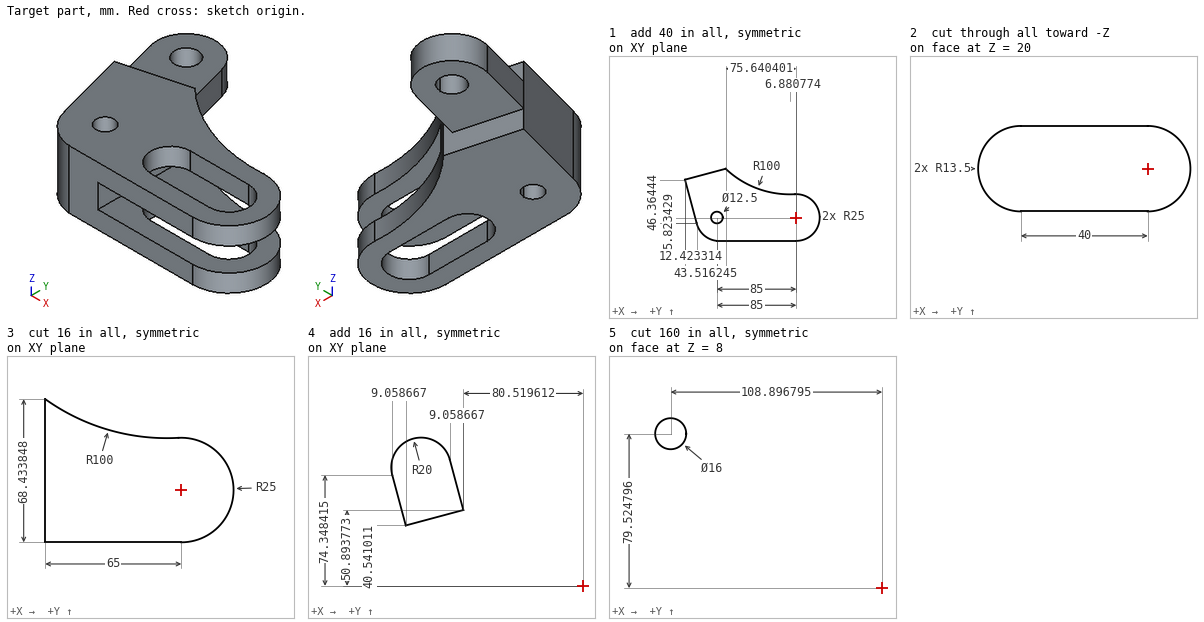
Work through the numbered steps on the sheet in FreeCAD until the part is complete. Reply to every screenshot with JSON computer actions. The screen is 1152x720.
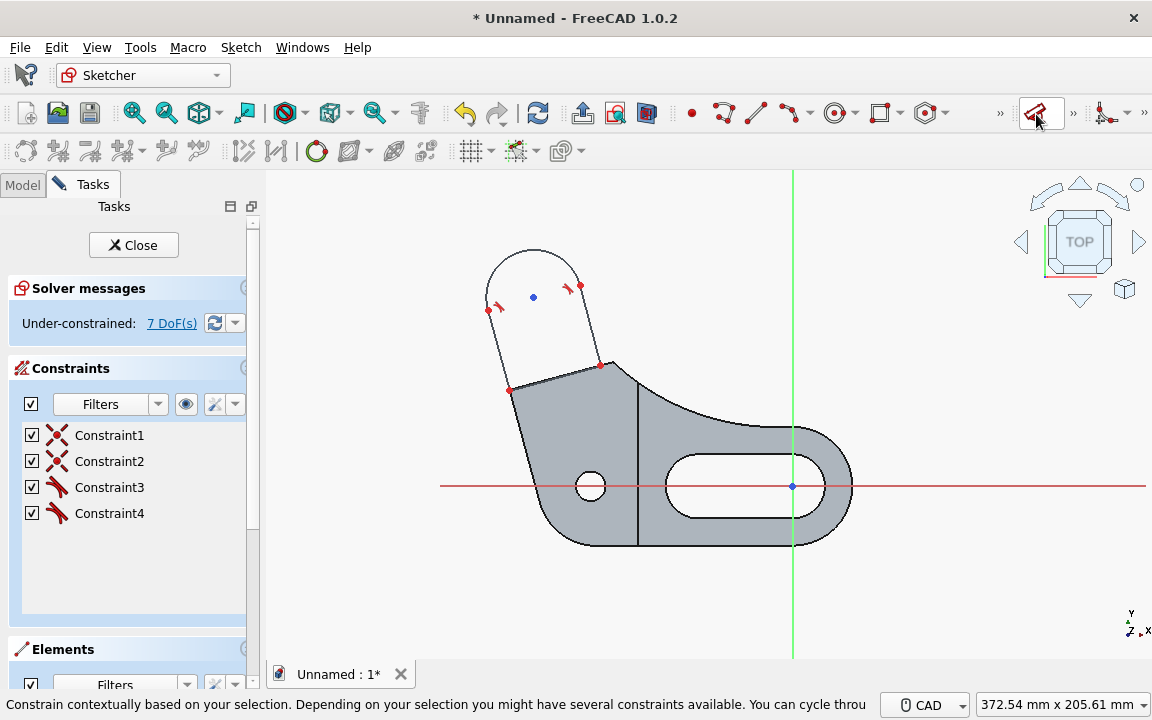
{"action": "left_click", "coordinate": [551, 253]}
{"action": "left_click", "coordinate": [562, 223]}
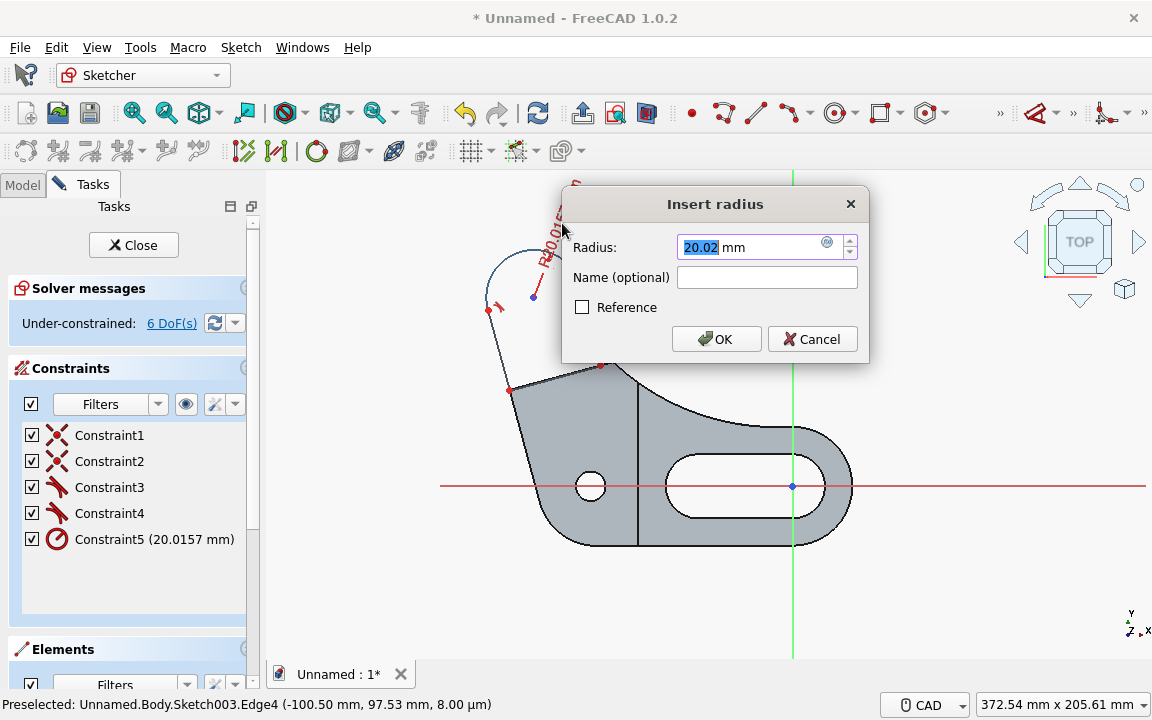
{"action": "type", "text": "20"}
{"action": "key", "text": "Return"}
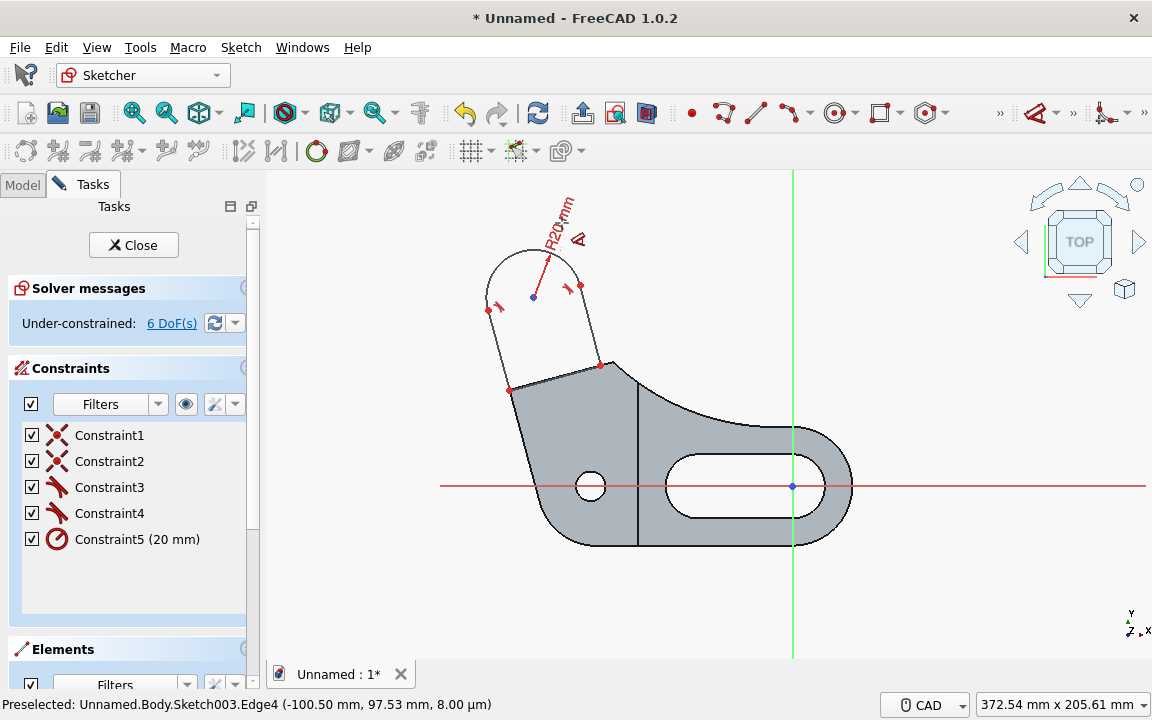
{"action": "scroll", "coordinate": [495, 334], "scroll_direction": "up", "scroll_amount": 4}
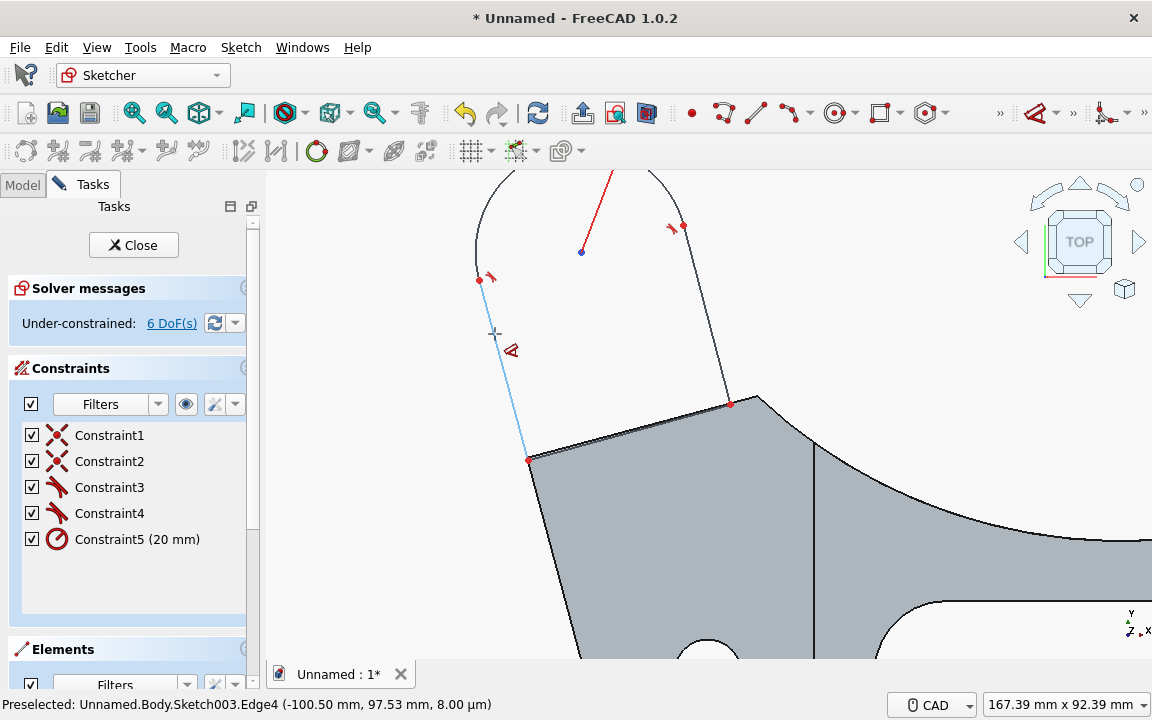
{"action": "left_click", "coordinate": [494, 334]}
{"action": "left_click", "coordinate": [504, 246]}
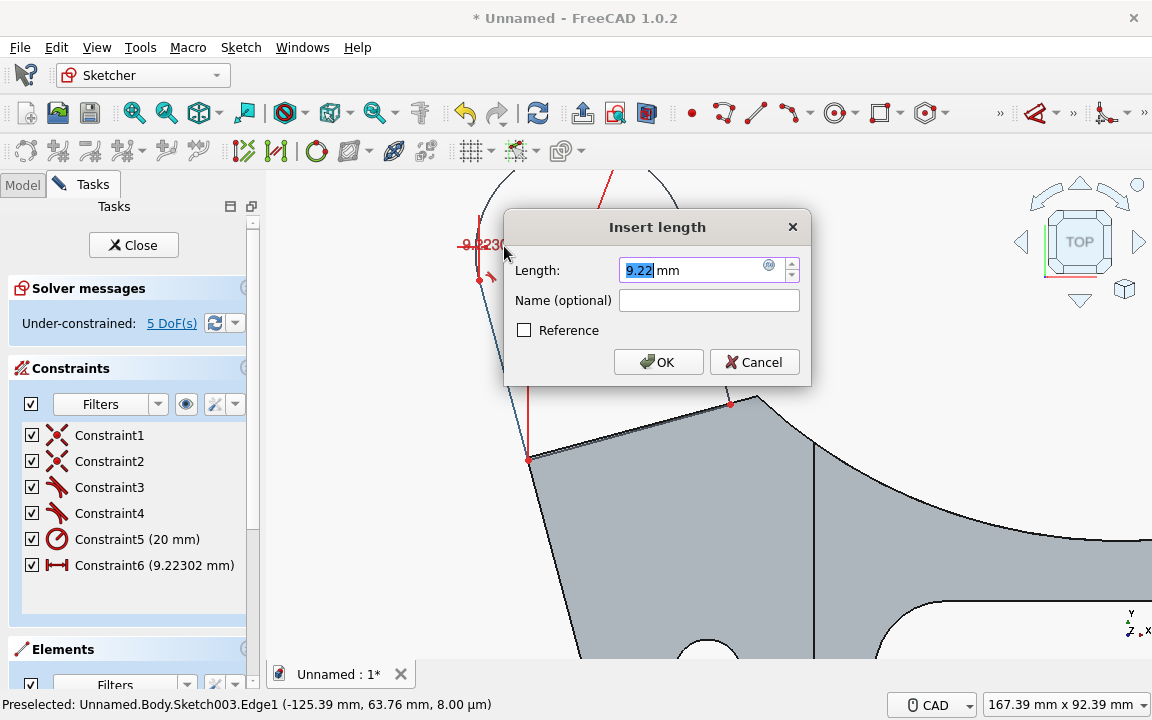
{"action": "type", "text": "9.058667"}
{"action": "key", "text": "Return"}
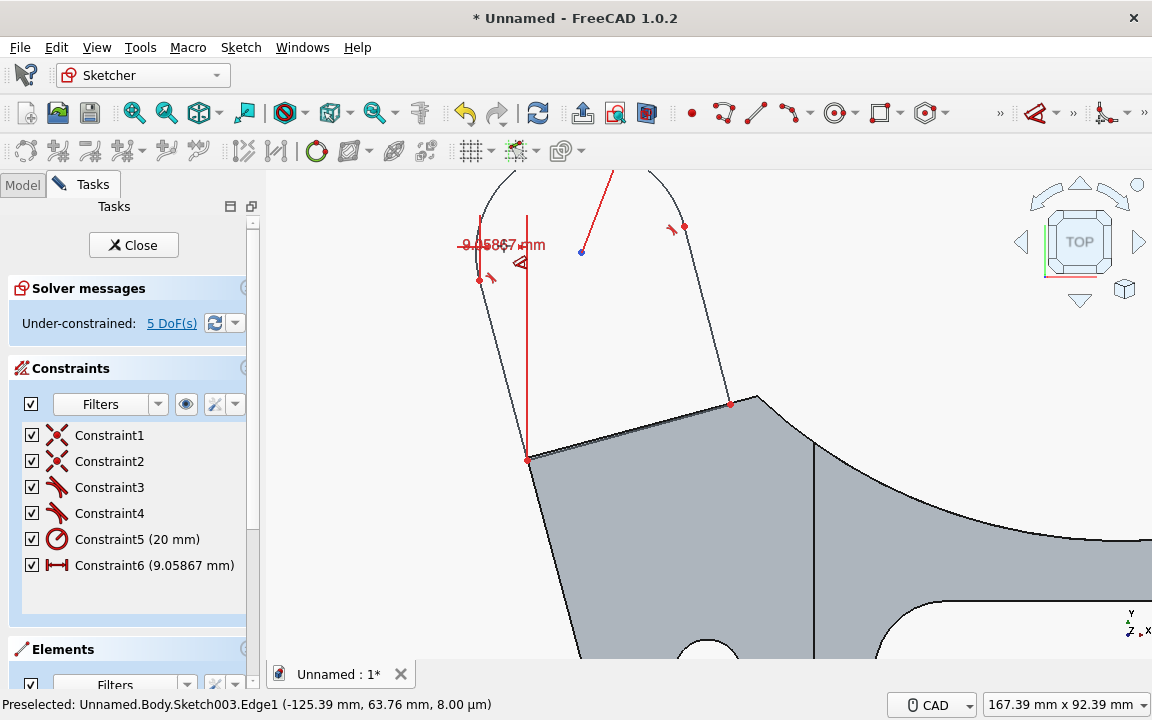
{"action": "left_click", "coordinate": [717, 351]}
{"action": "left_click", "coordinate": [707, 439]}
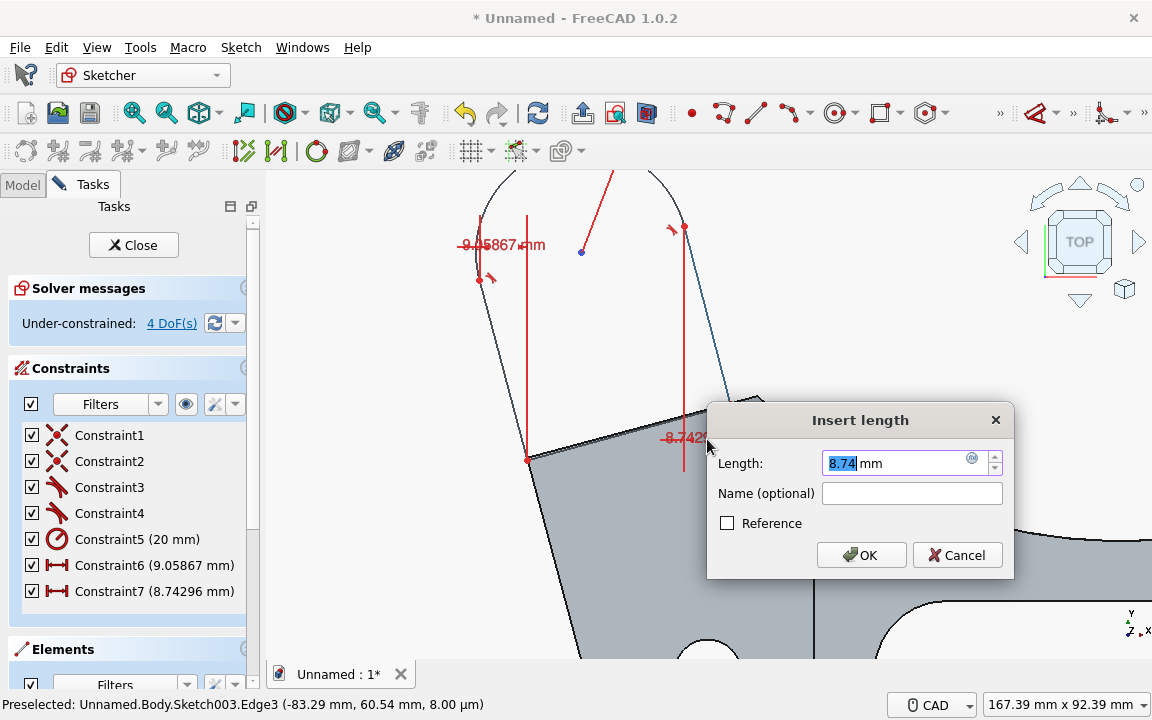
{"action": "type", "text": "9.058667"}
{"action": "key", "text": "Return"}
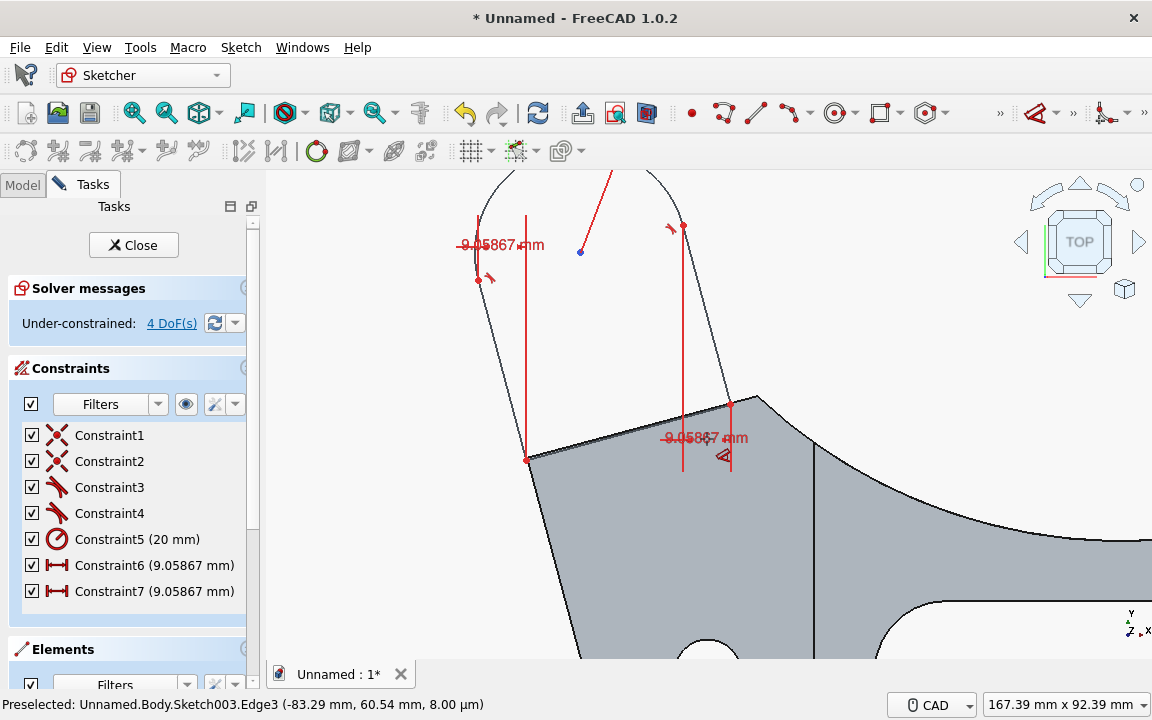
{"action": "left_click", "coordinate": [478, 280]}
{"action": "left_click", "coordinate": [444, 456]}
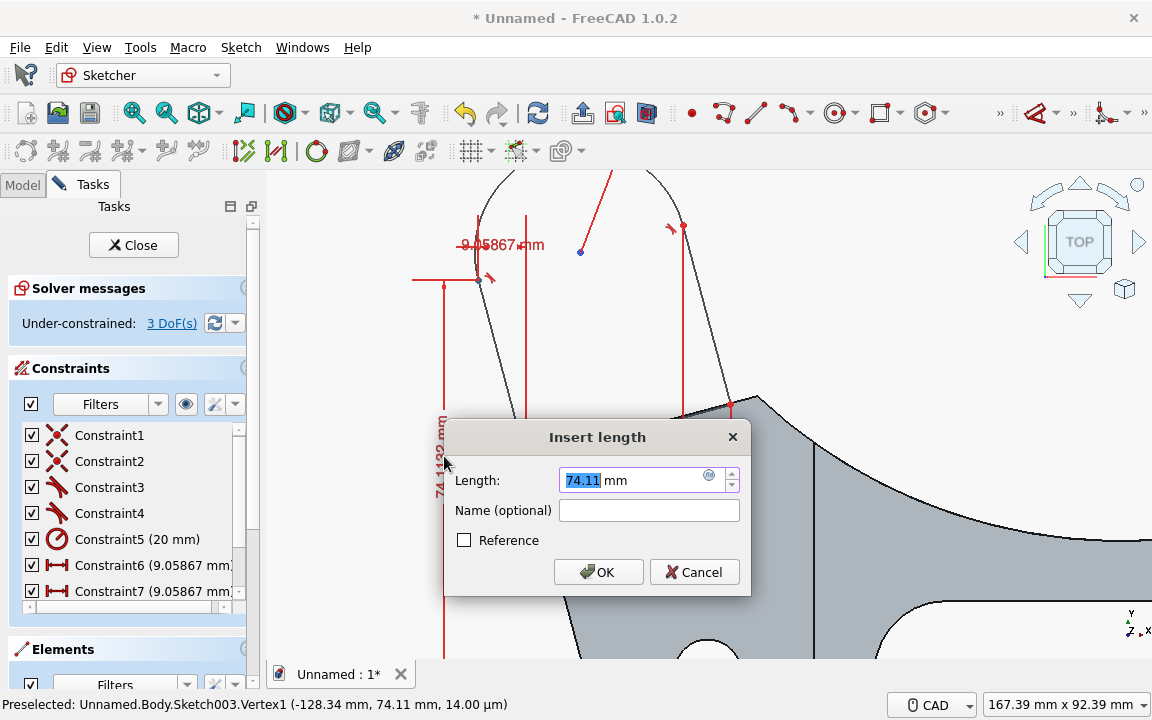
{"action": "type", "text": "74.348415"}
{"action": "key", "text": "Return"}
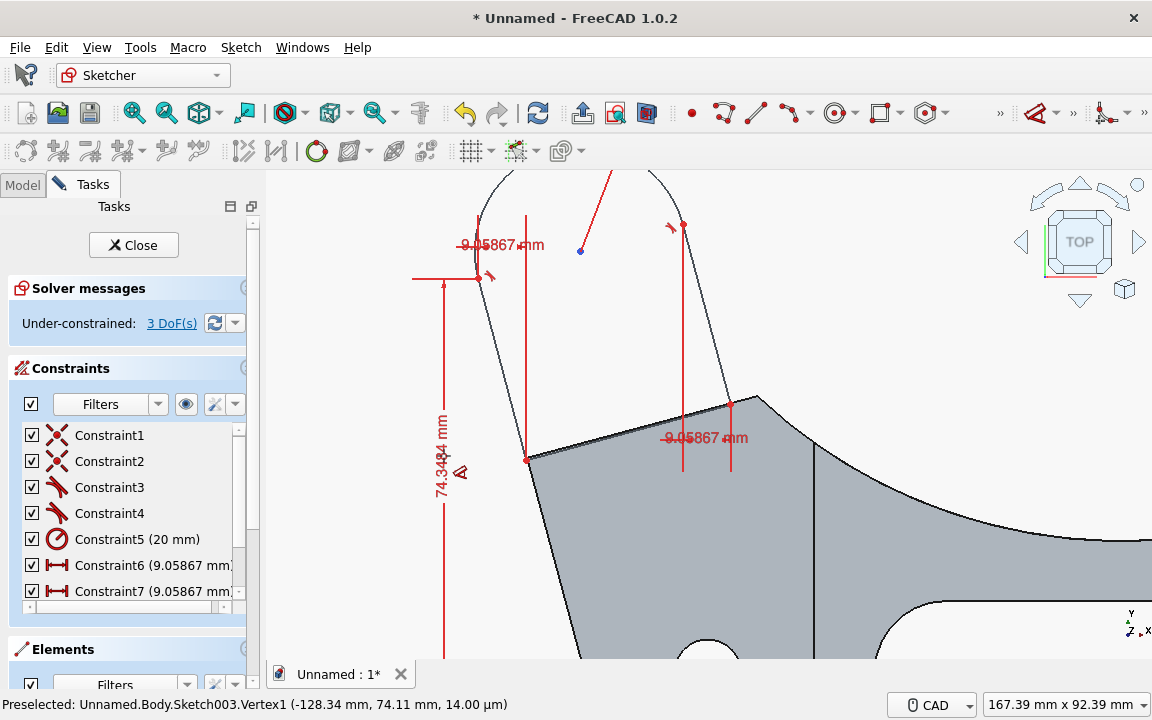
{"action": "left_click", "coordinate": [526, 460]}
{"action": "left_click", "coordinate": [492, 546]}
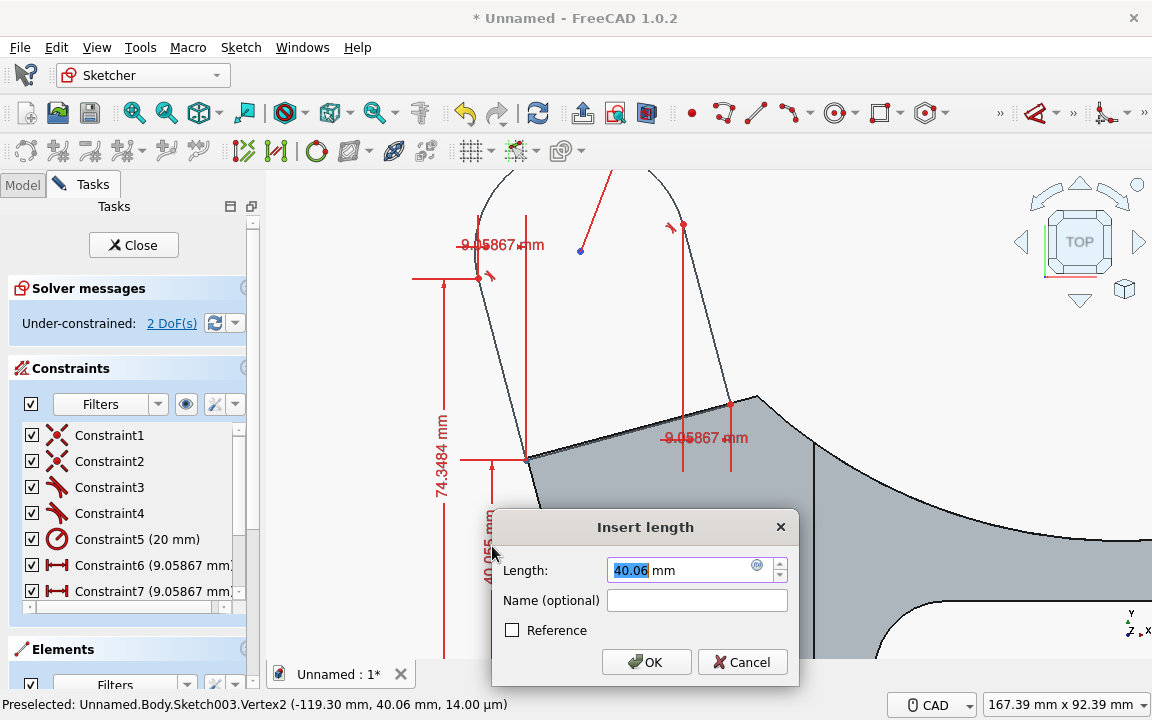
{"action": "type", "text": "40.541011"}
{"action": "key", "text": "Return"}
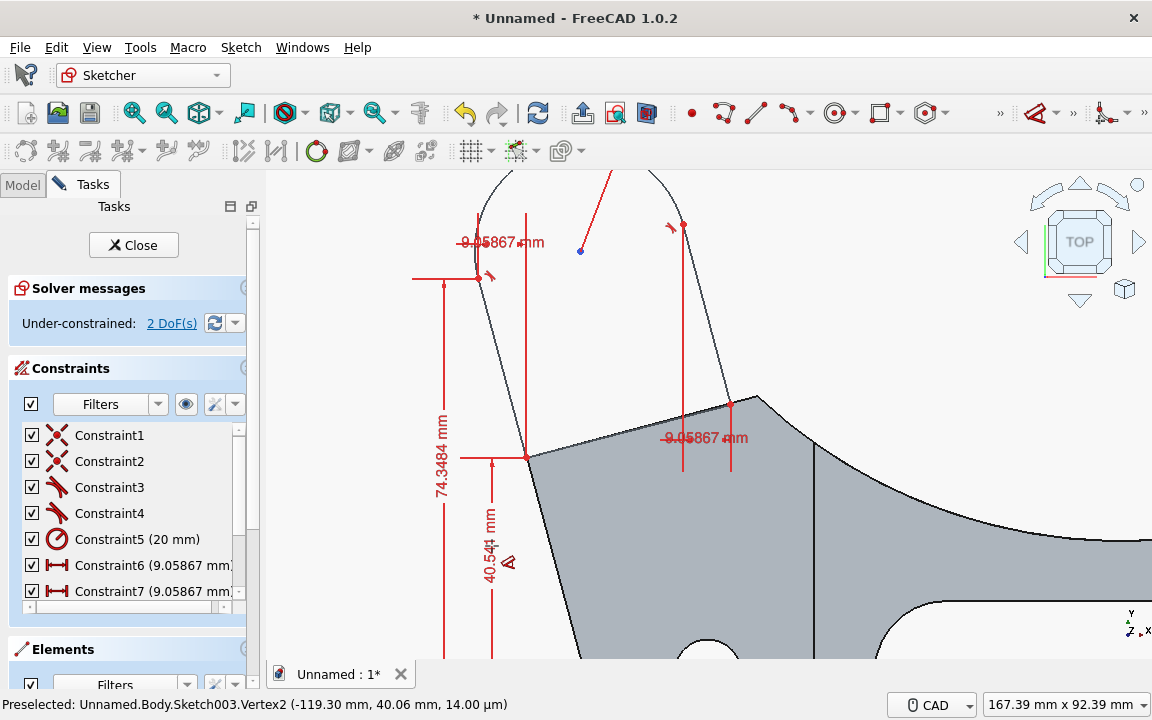
{"action": "left_click", "coordinate": [731, 405]}
{"action": "left_click", "coordinate": [859, 371]}